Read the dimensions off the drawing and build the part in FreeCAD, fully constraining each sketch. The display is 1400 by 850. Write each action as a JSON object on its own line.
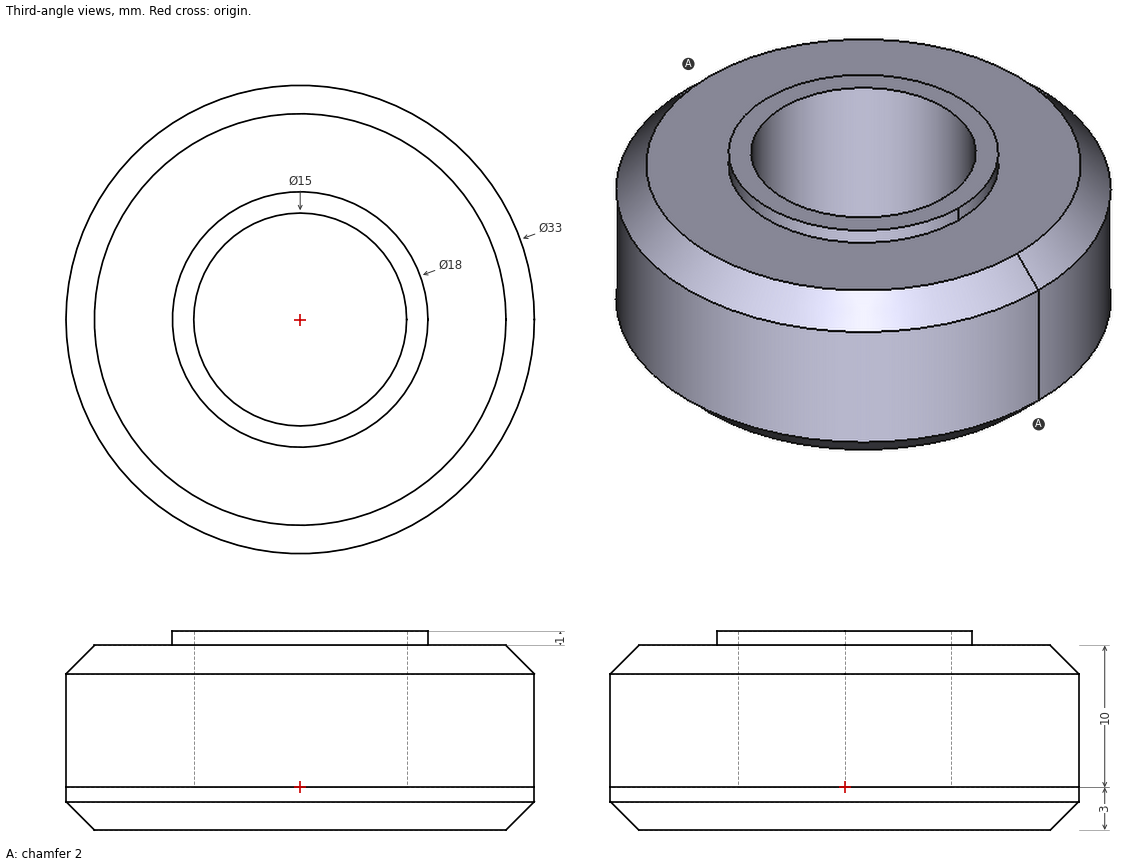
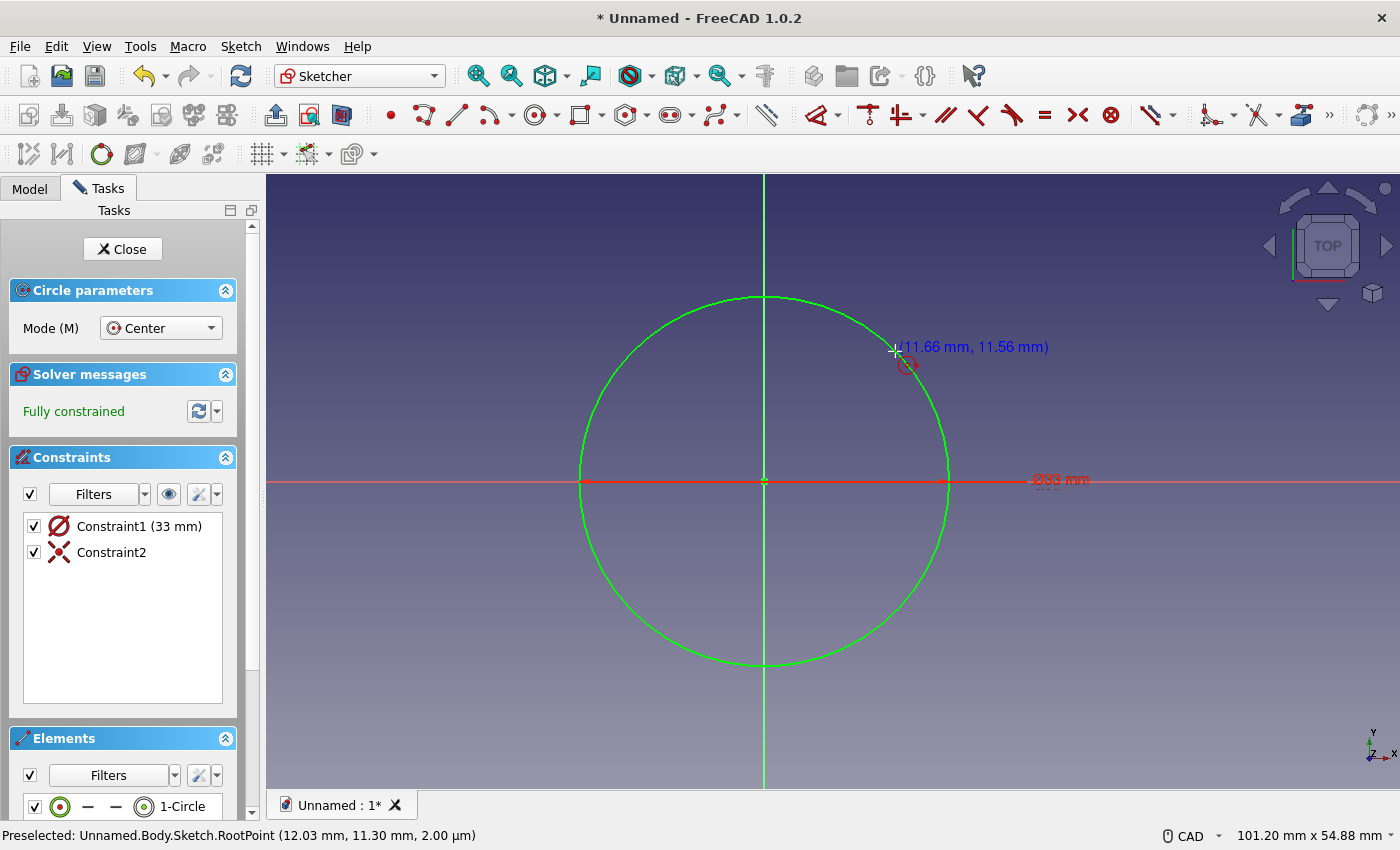
{"action": "left_click", "coordinate": [764, 482]}
{"action": "mouse_move", "coordinate": [824, 422]}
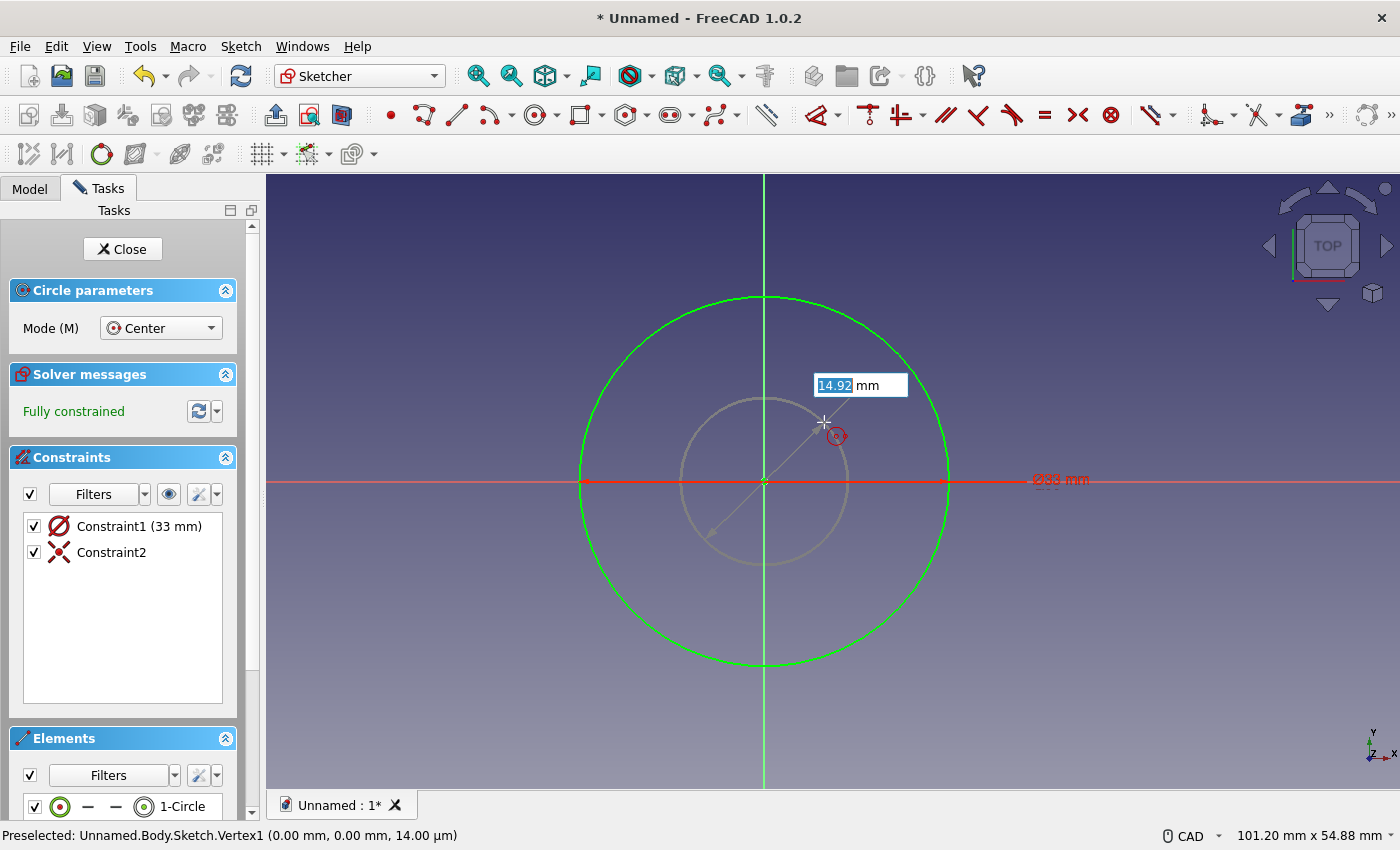
{"action": "type", "text": "15"}
{"action": "key", "text": "Return"}
{"action": "key", "text": "Escape"}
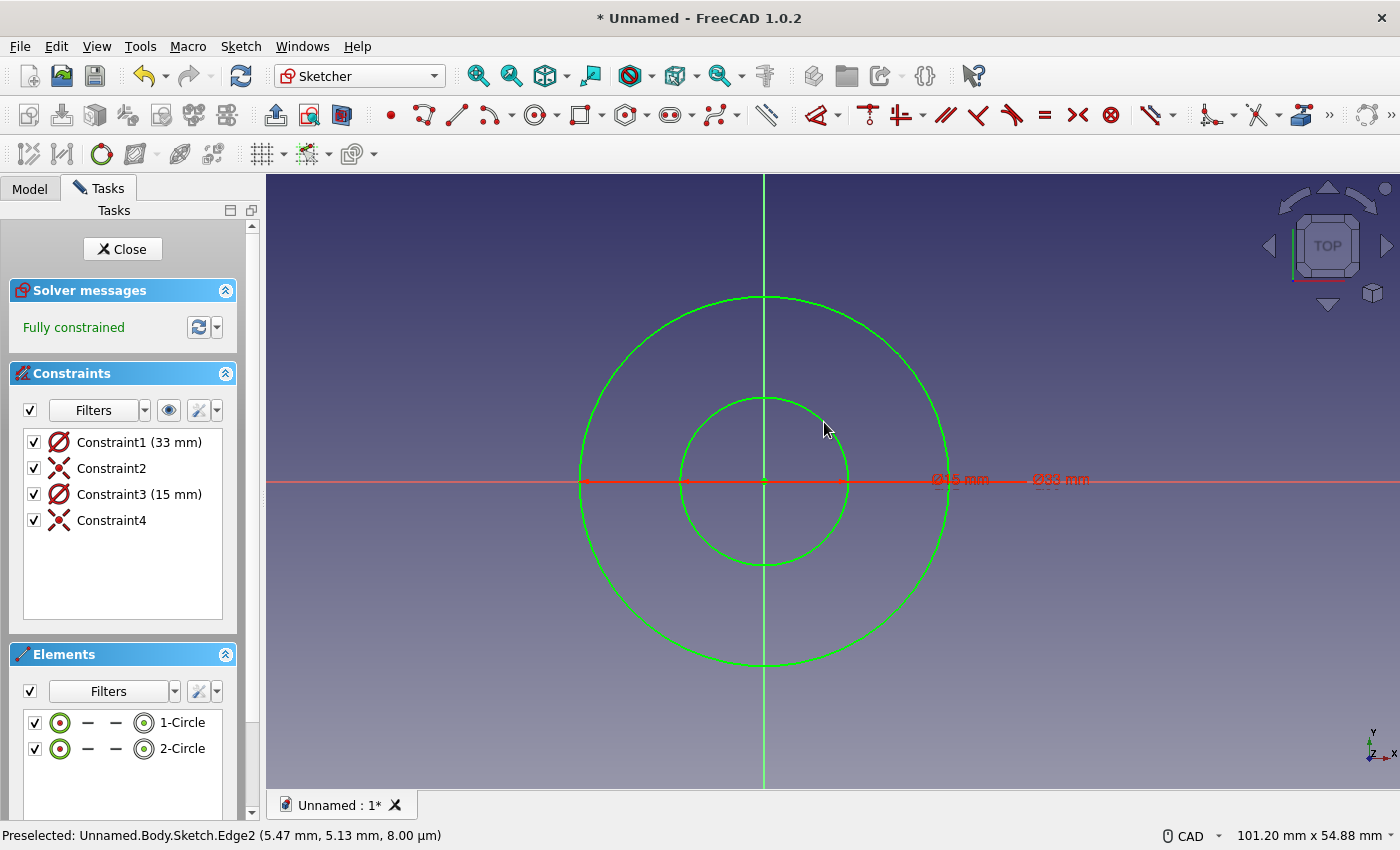
{"action": "left_click", "coordinate": [123, 249]}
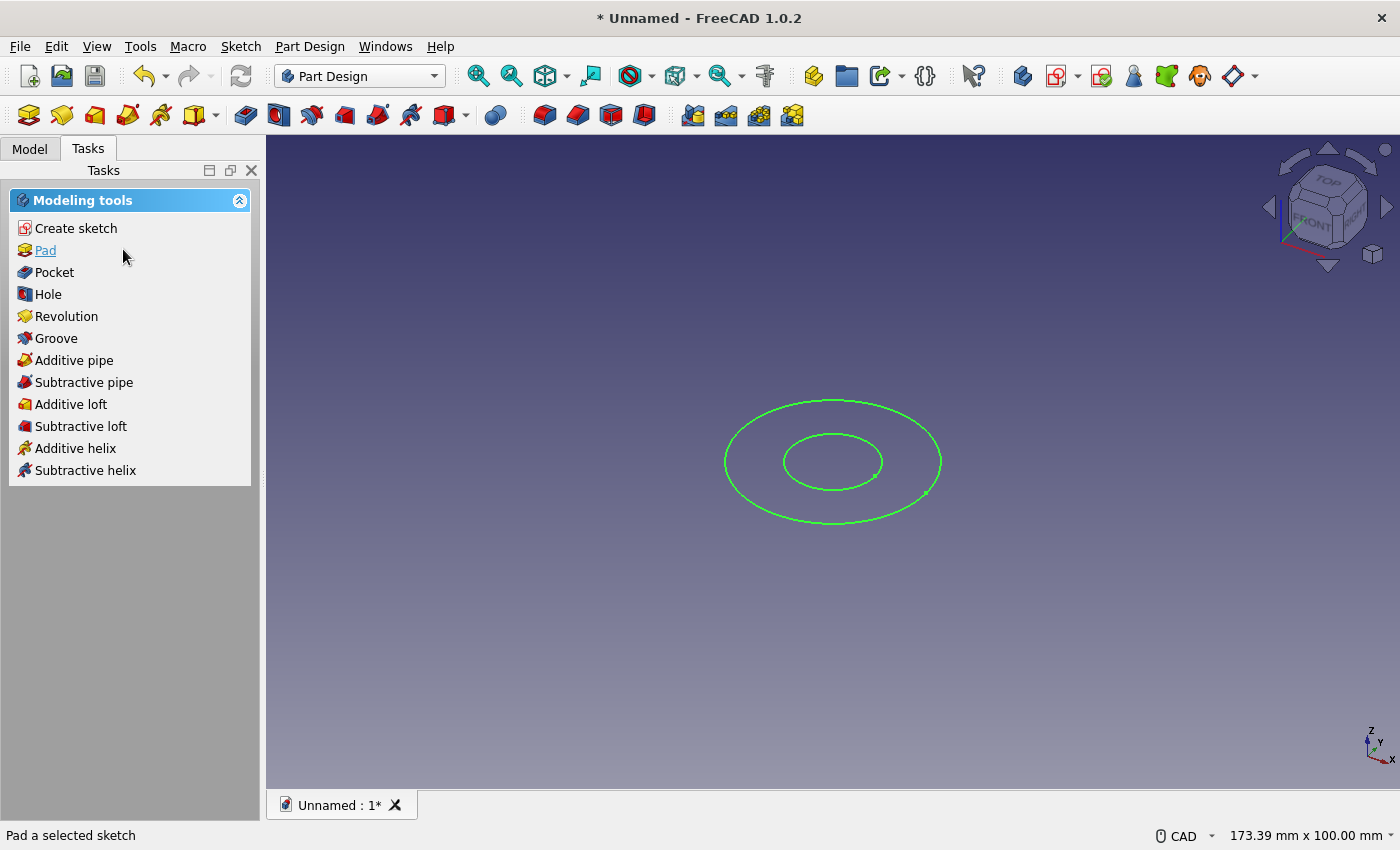
{"action": "left_click", "coordinate": [29, 116]}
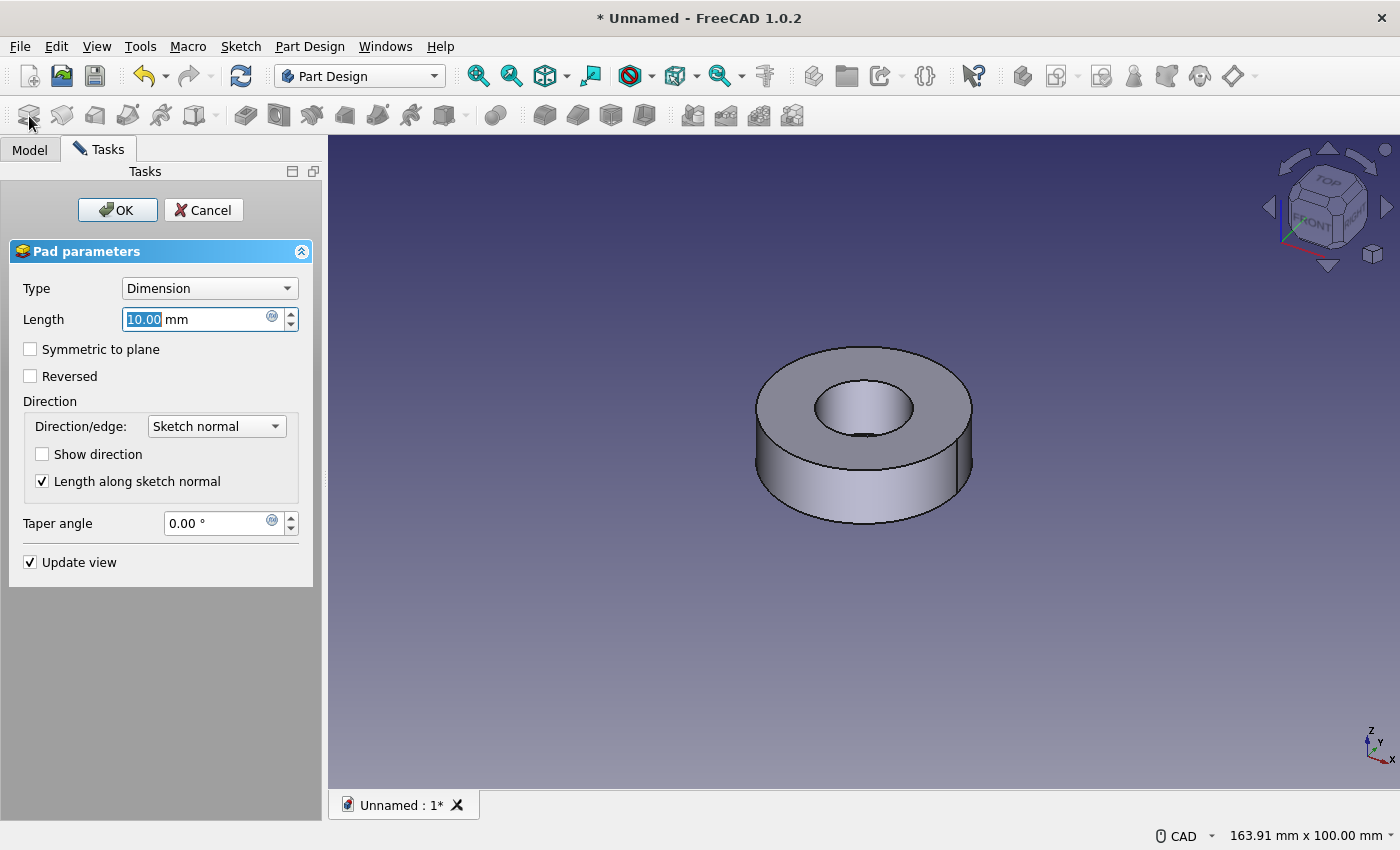
{"action": "type", "text": "10"}
{"action": "key", "text": "Tab"}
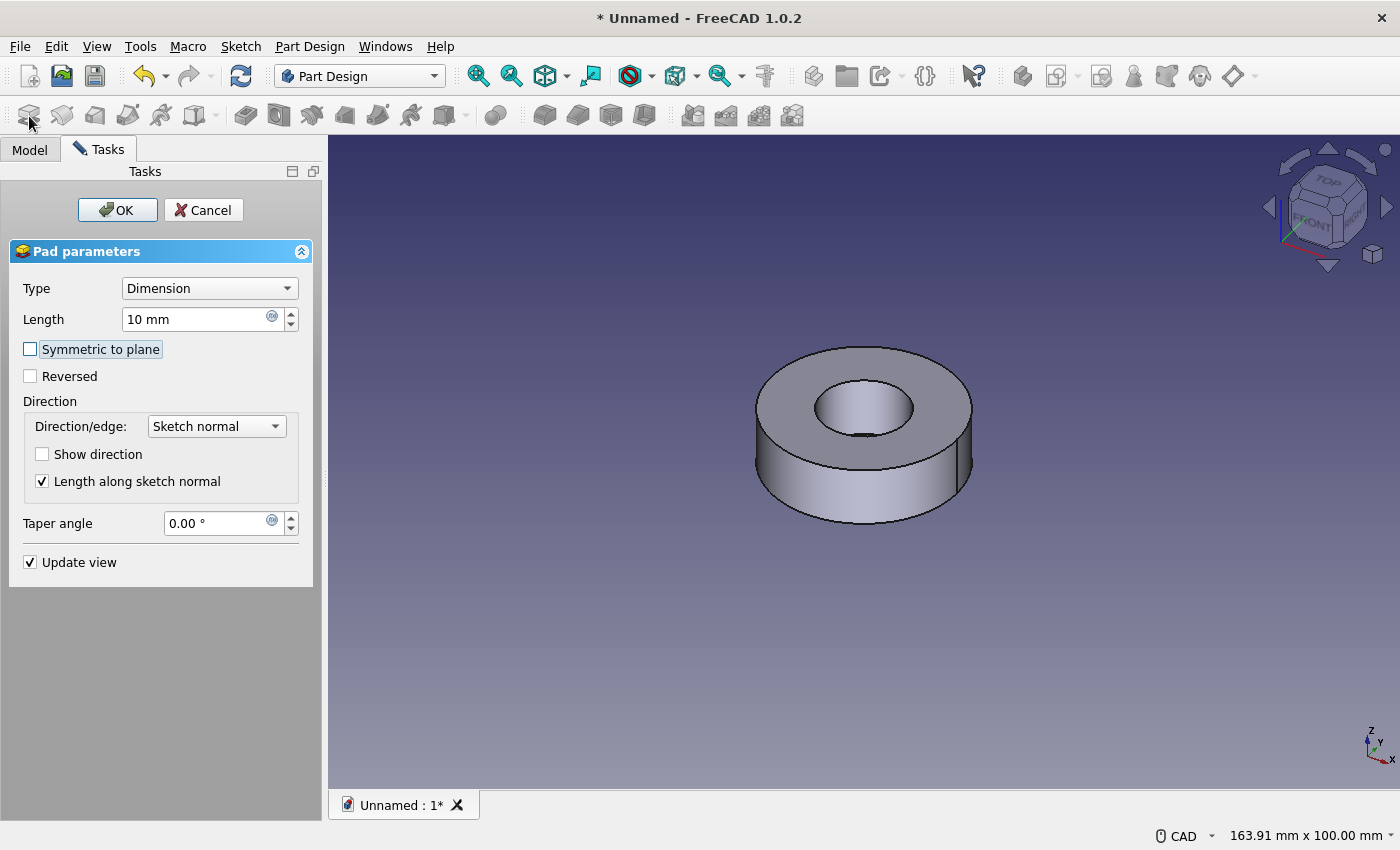
{"action": "left_click", "coordinate": [118, 210]}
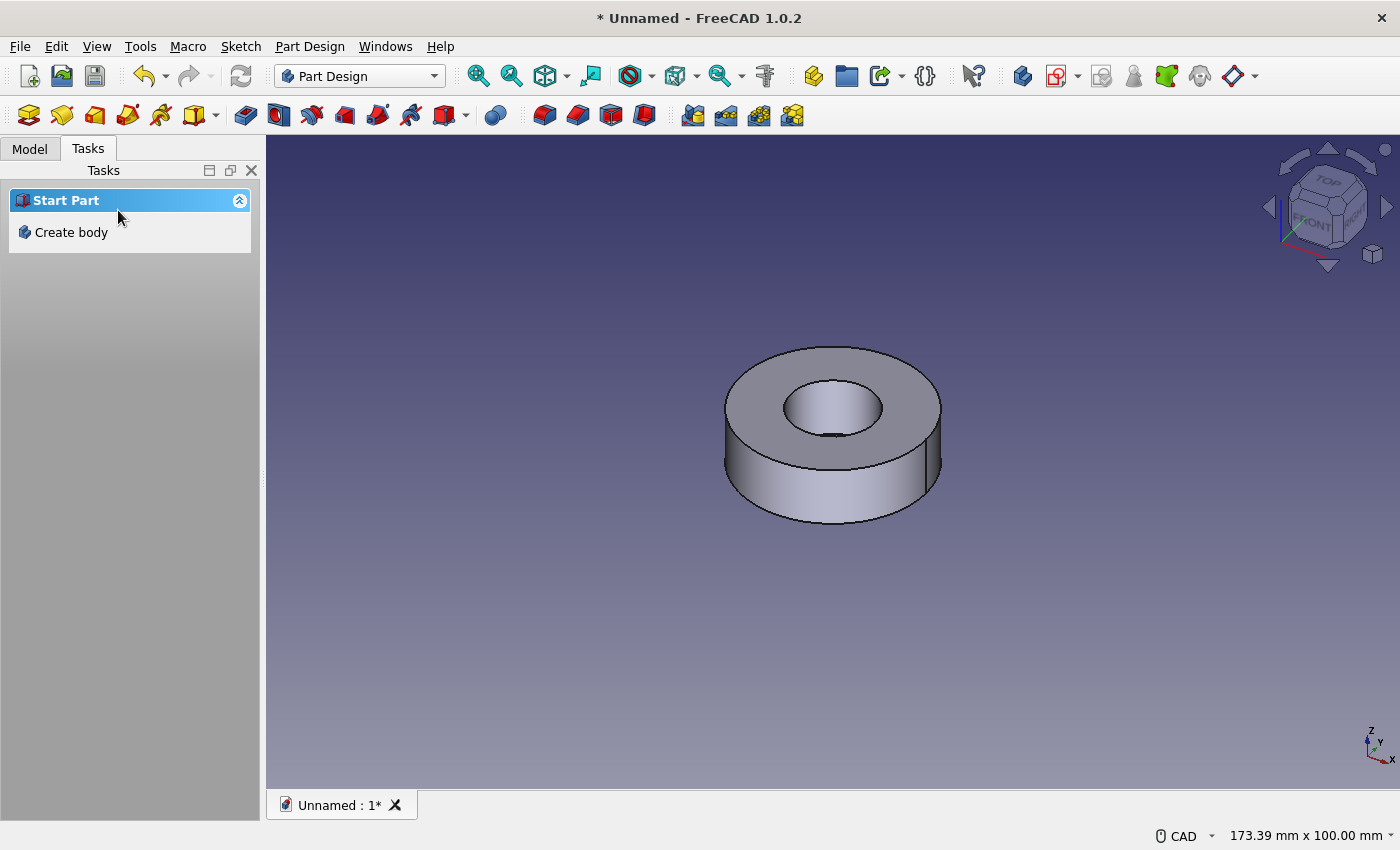
{"action": "key", "text": "v f"}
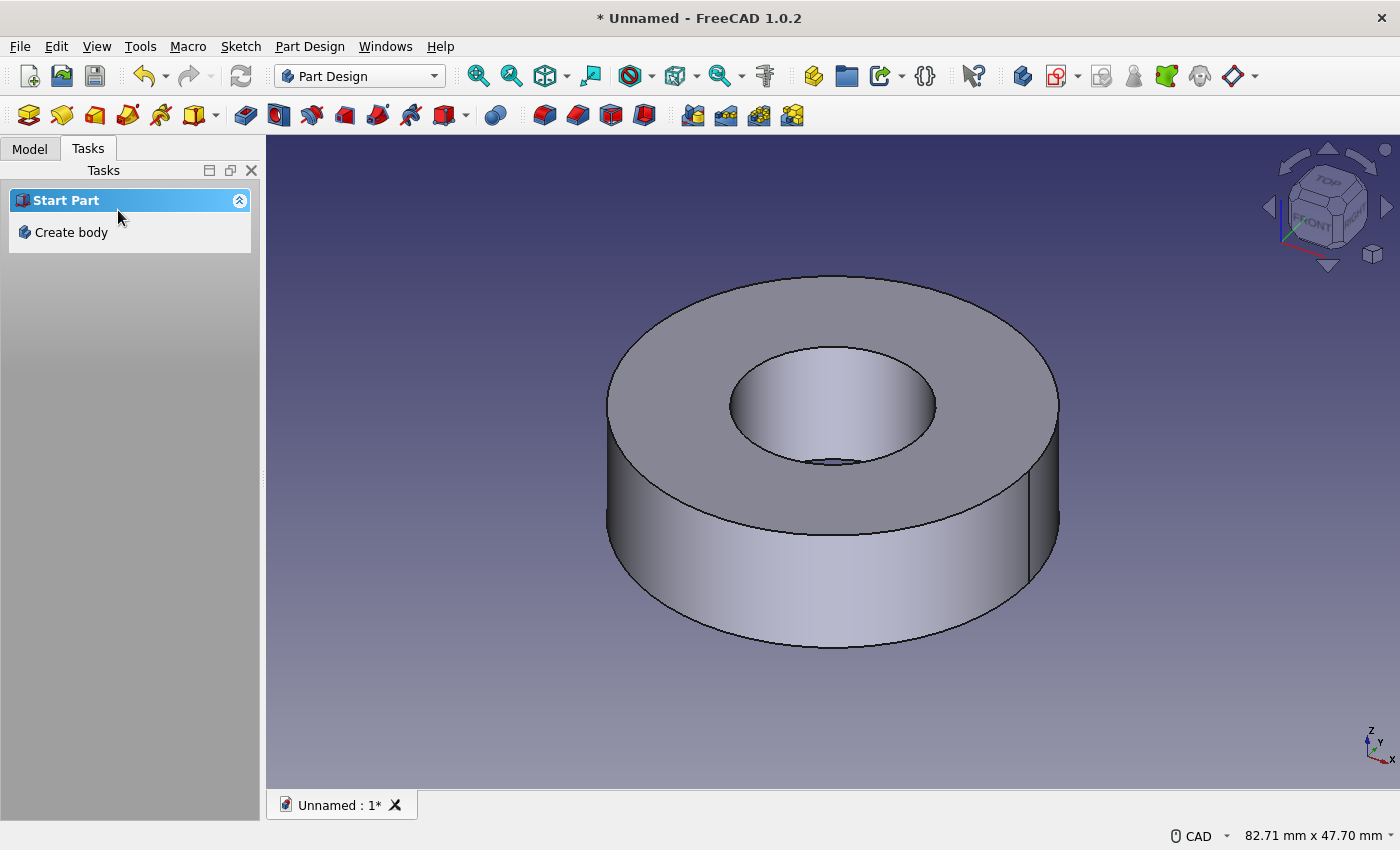
{"action": "left_click", "coordinate": [1009, 378]}